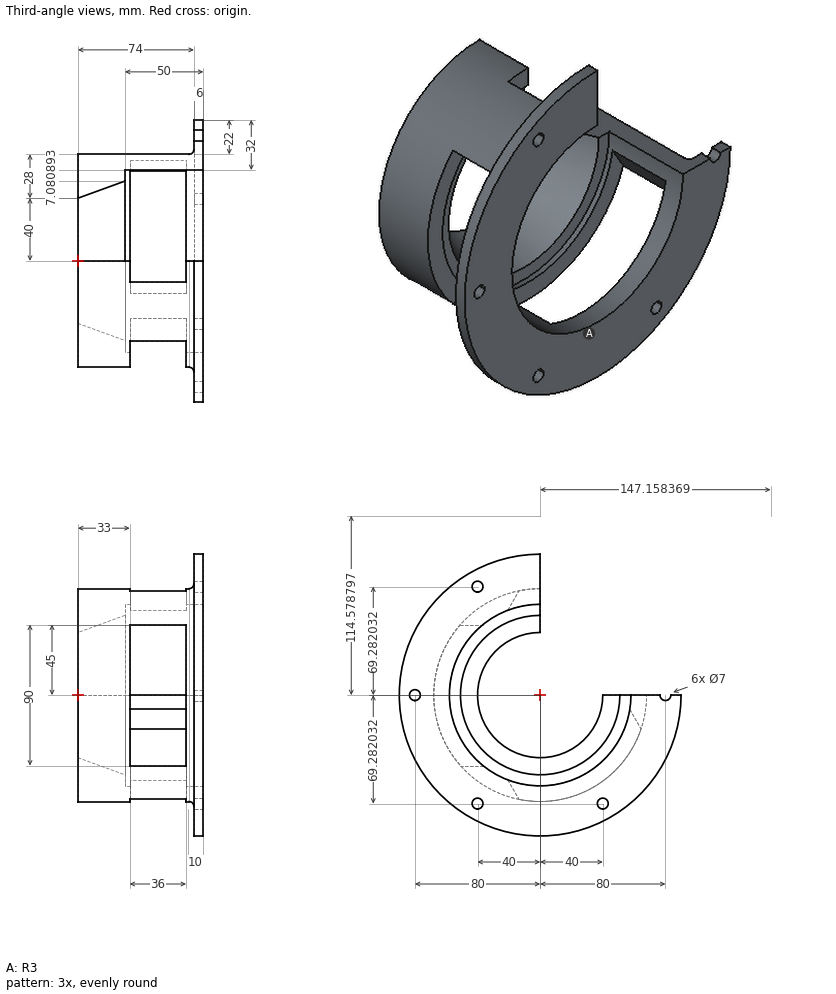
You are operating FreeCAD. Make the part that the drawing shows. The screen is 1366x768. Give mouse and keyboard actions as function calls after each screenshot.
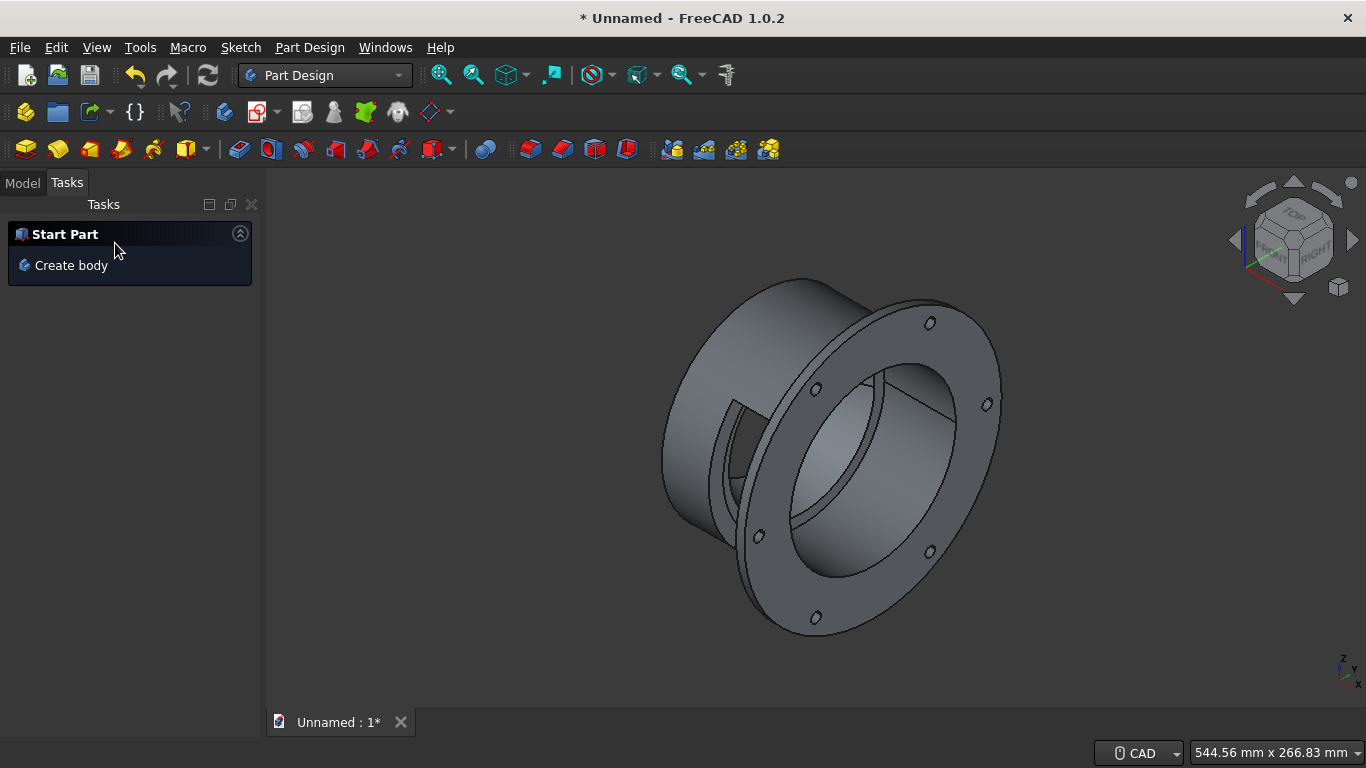
click(23, 182)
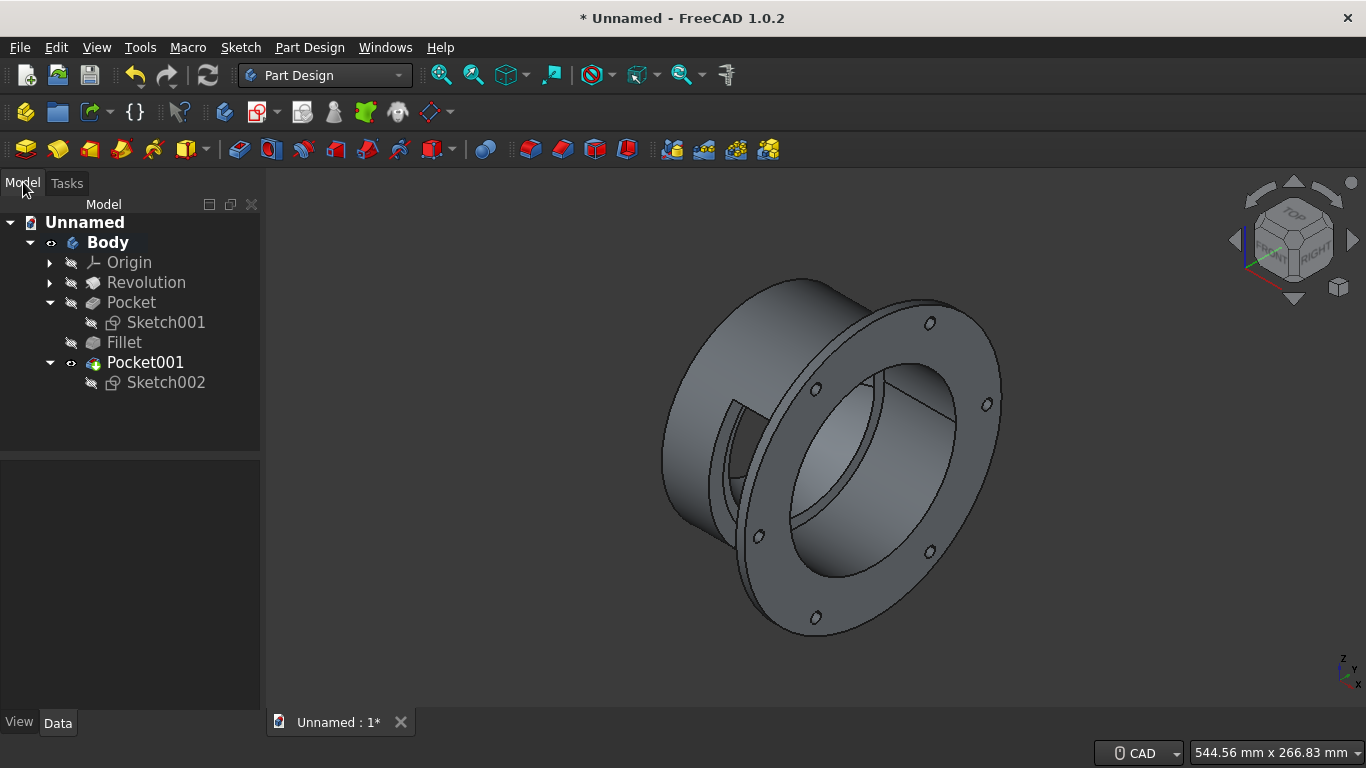
click(116, 363)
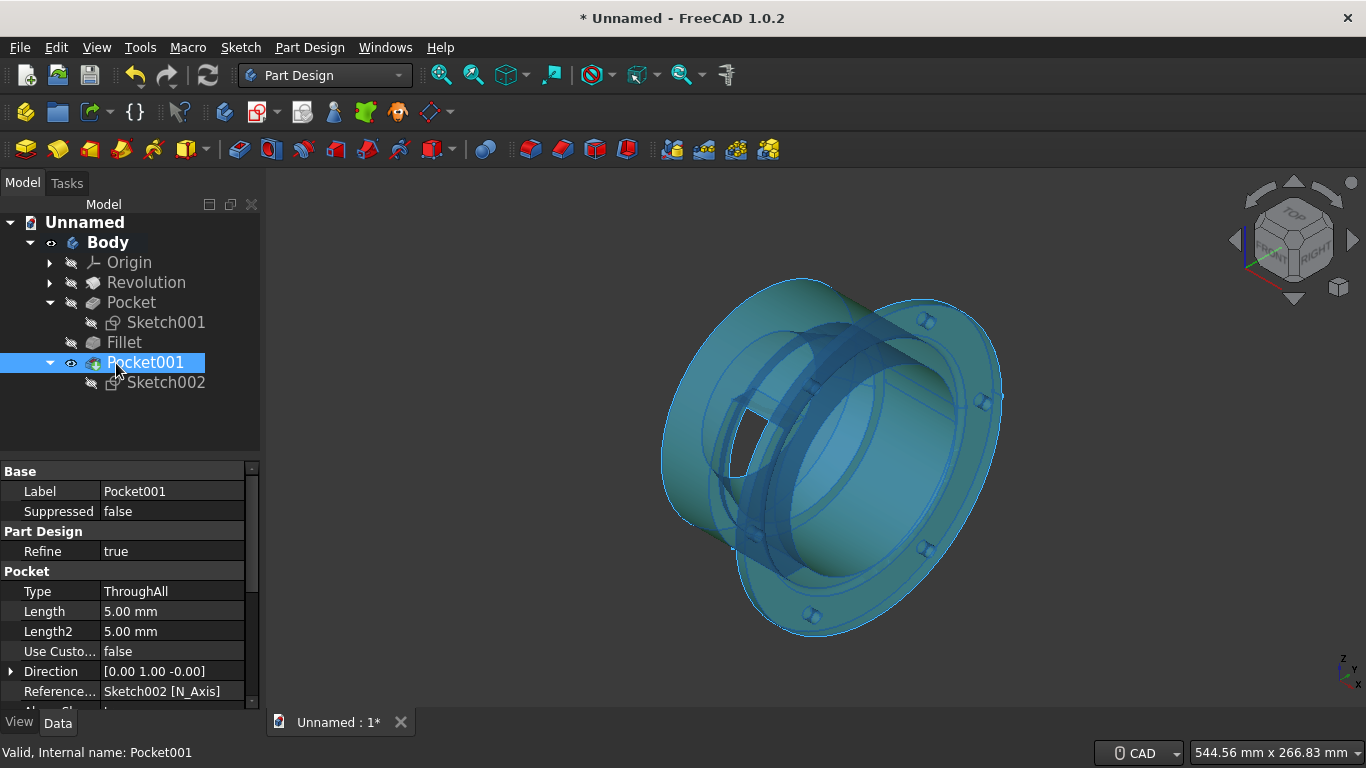
click(736, 150)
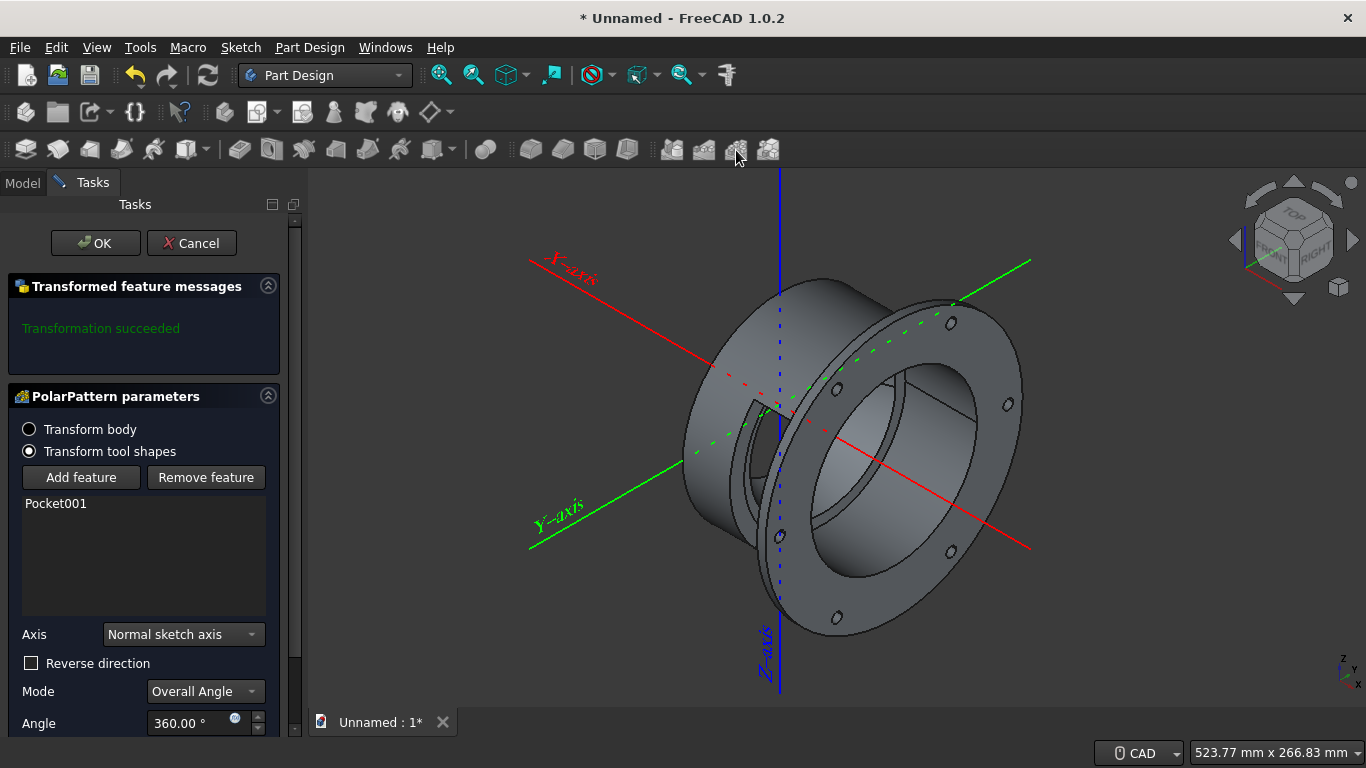
click(184, 634)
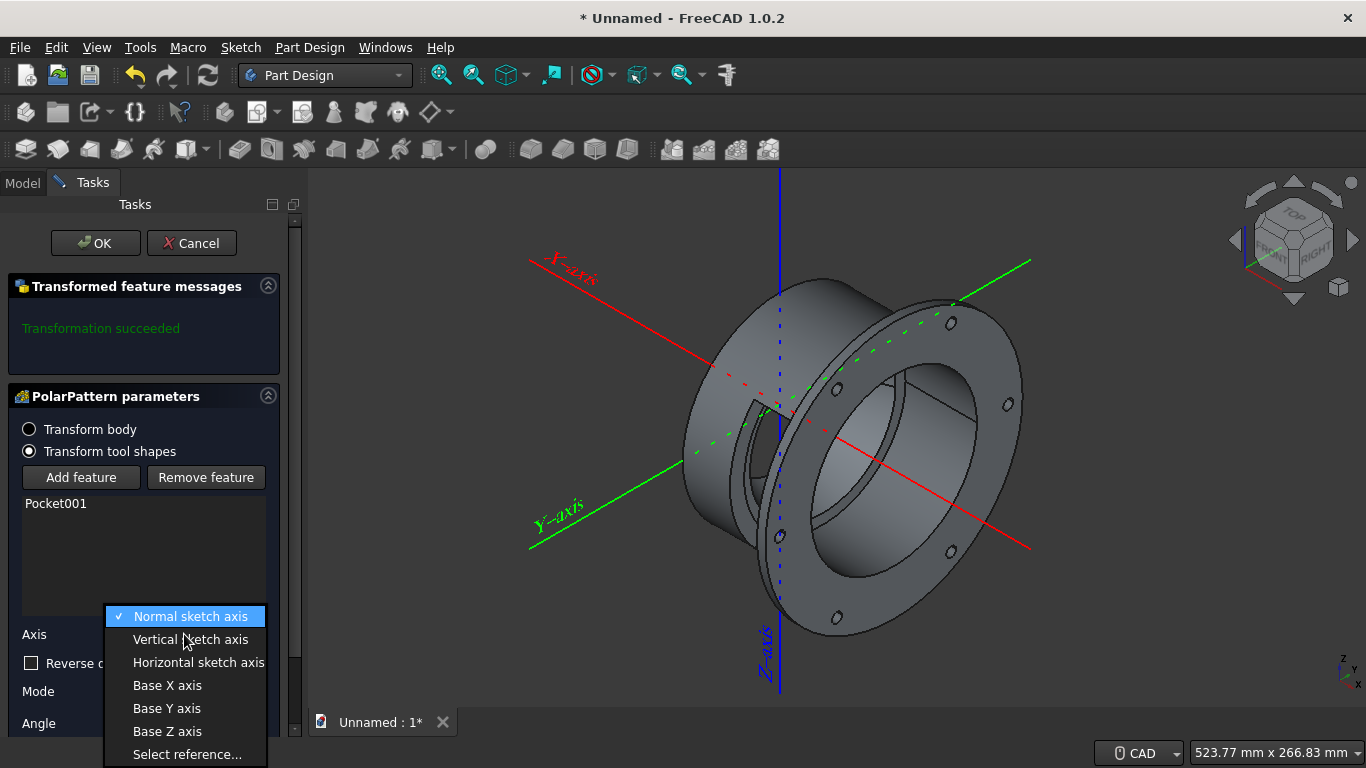
click(184, 686)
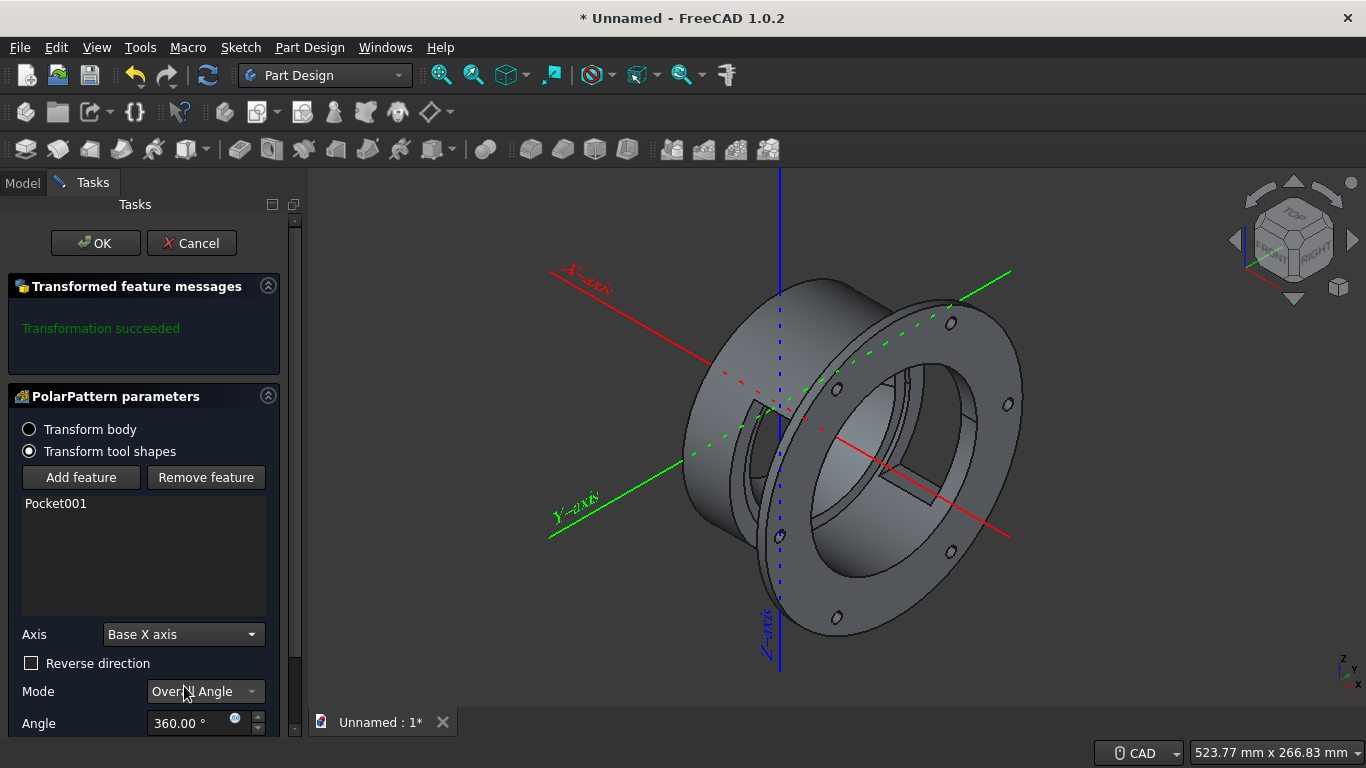
scroll(295, 475, down, 2)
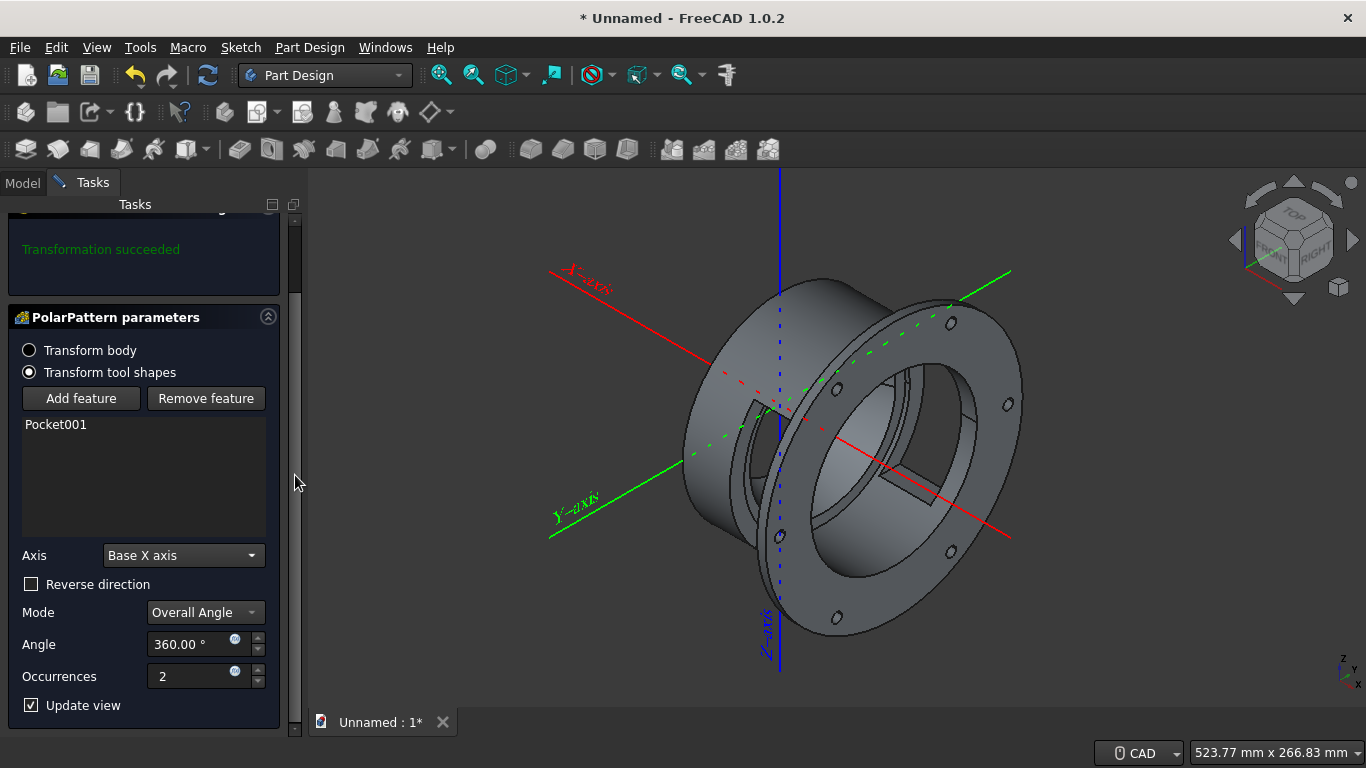
triple_click(198, 676)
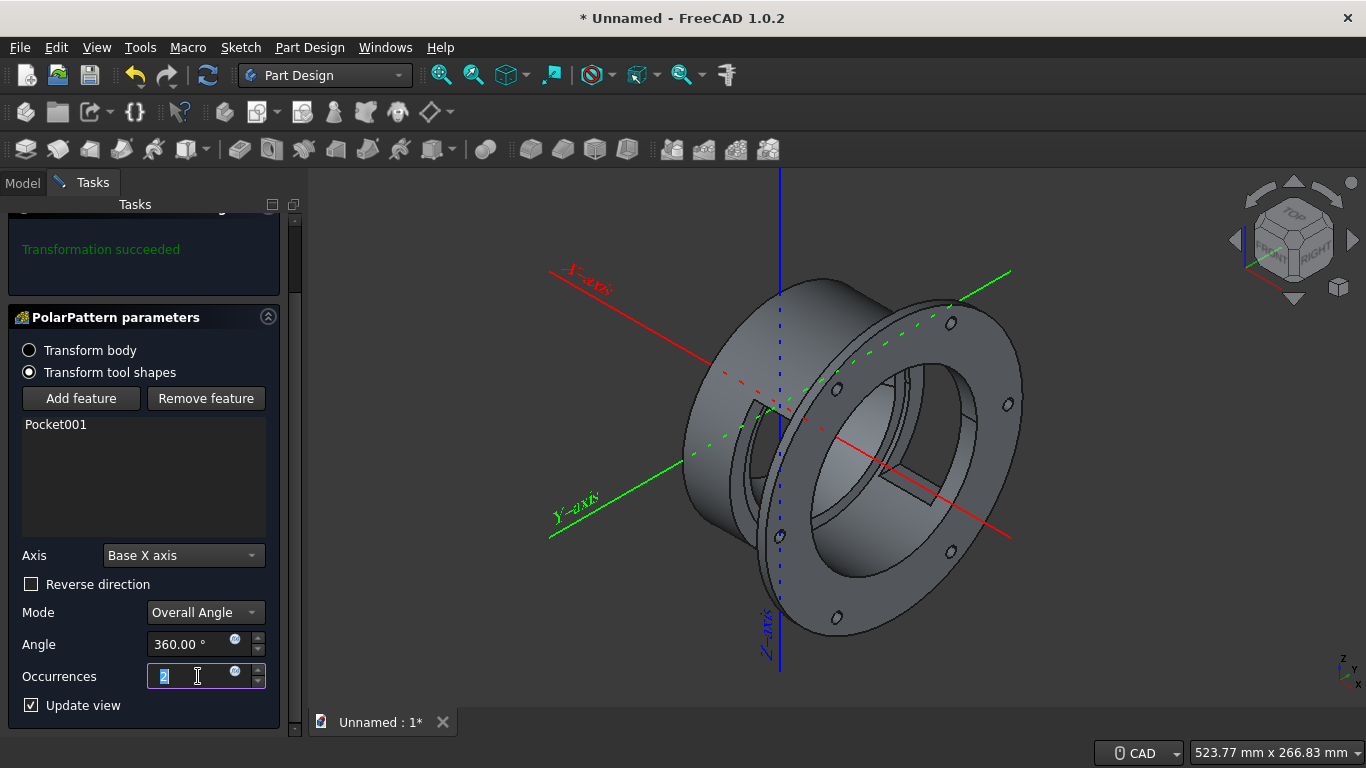
text(3)
key(Tab)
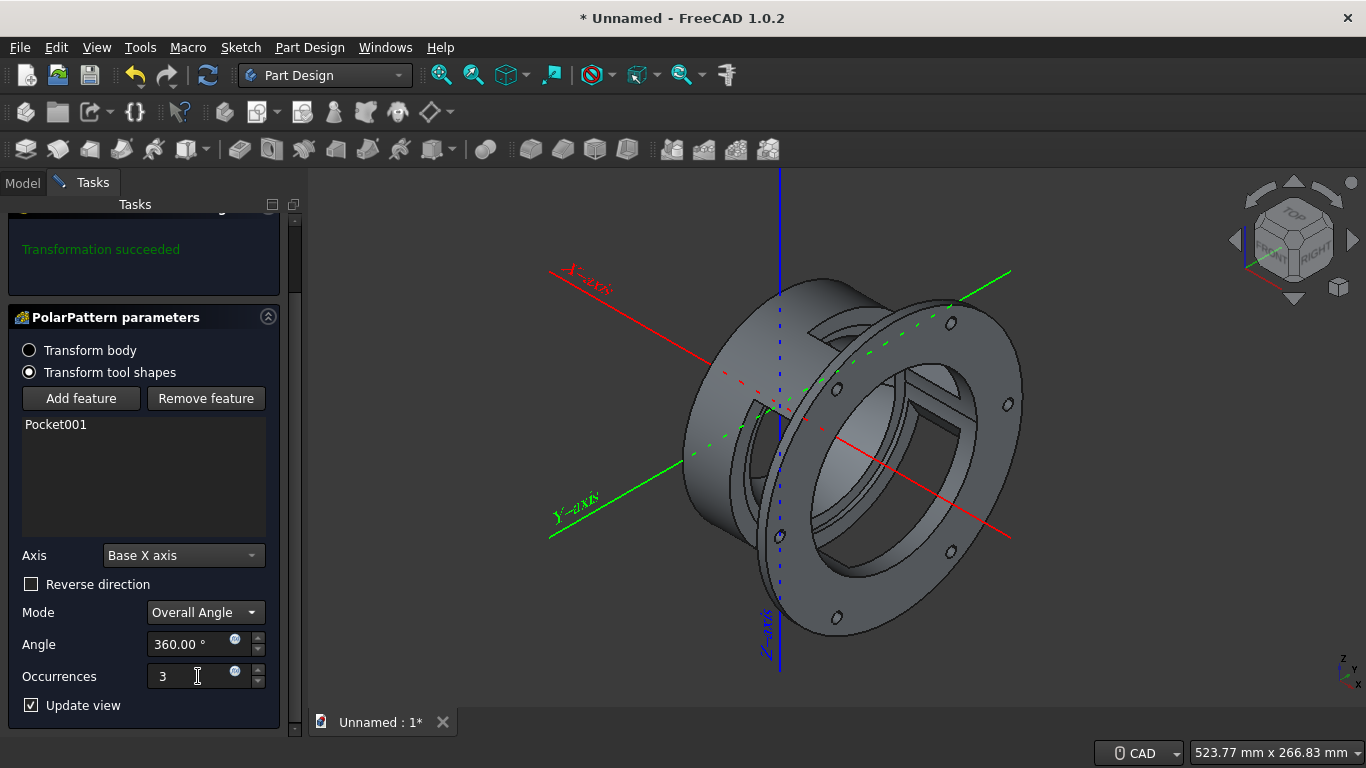
scroll(295, 475, up, 3)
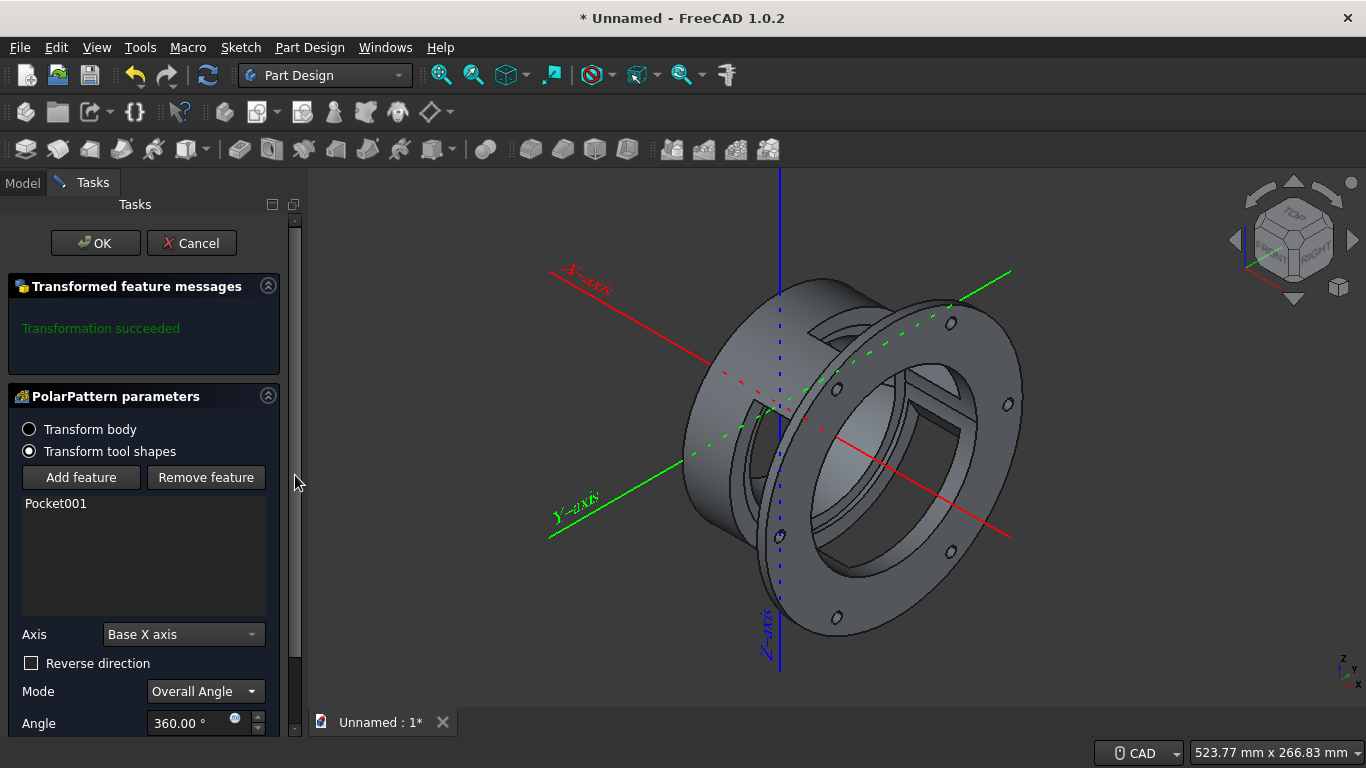
click(96, 243)